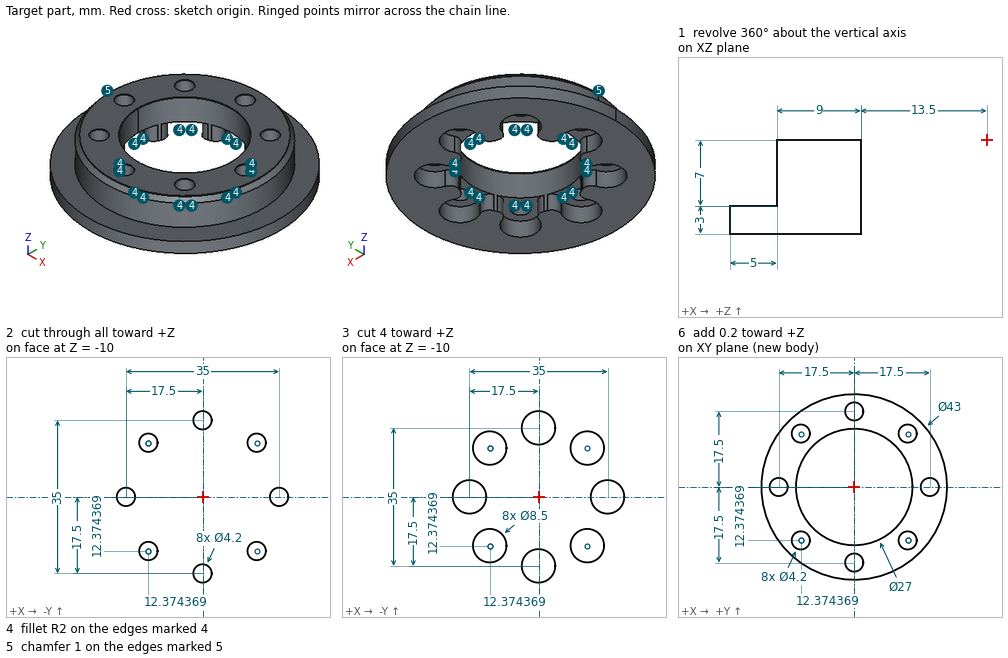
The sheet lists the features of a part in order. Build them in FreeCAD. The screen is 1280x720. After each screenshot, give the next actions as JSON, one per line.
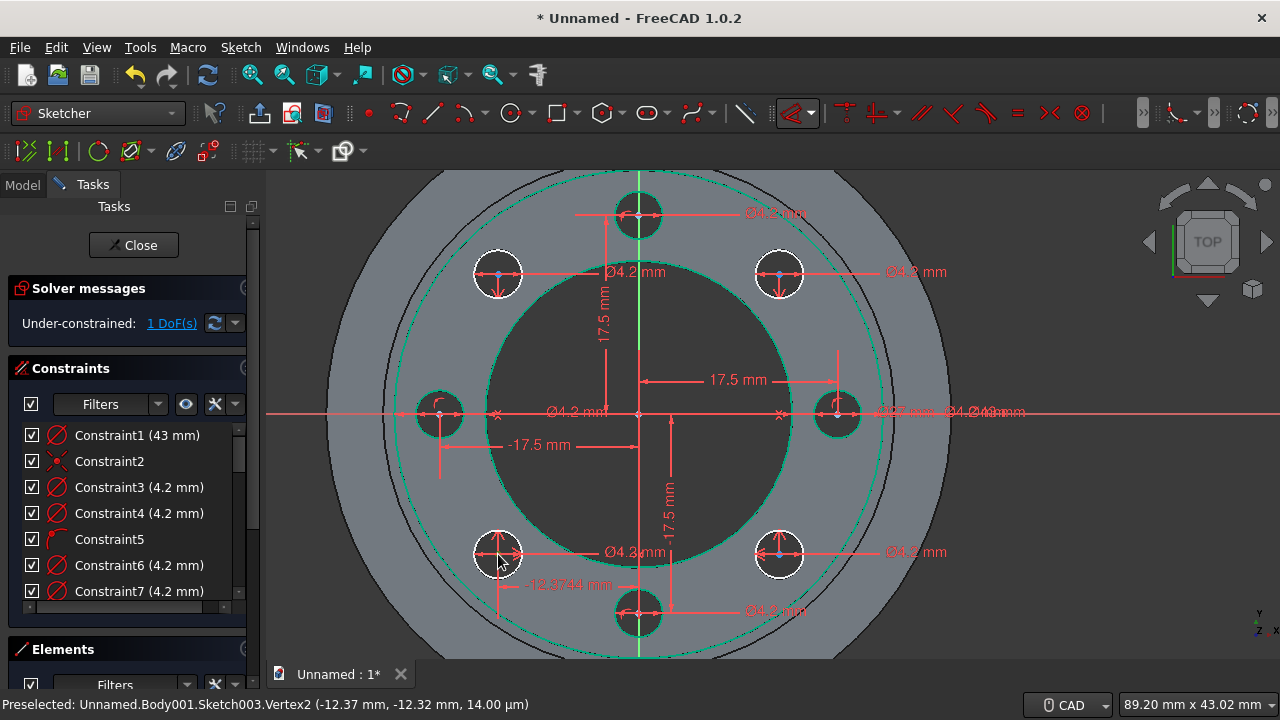
{"action": "key", "text": "i"}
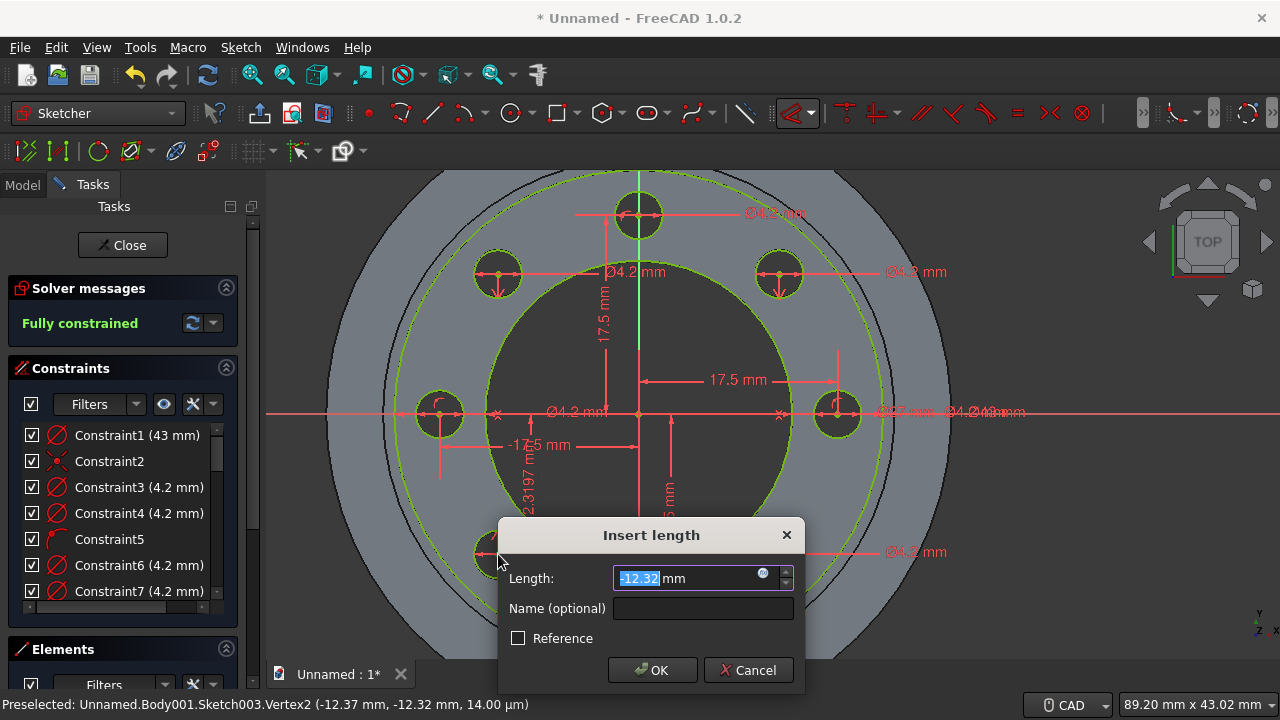
{"action": "type", "text": "-12.374369"}
{"action": "key", "text": "Return"}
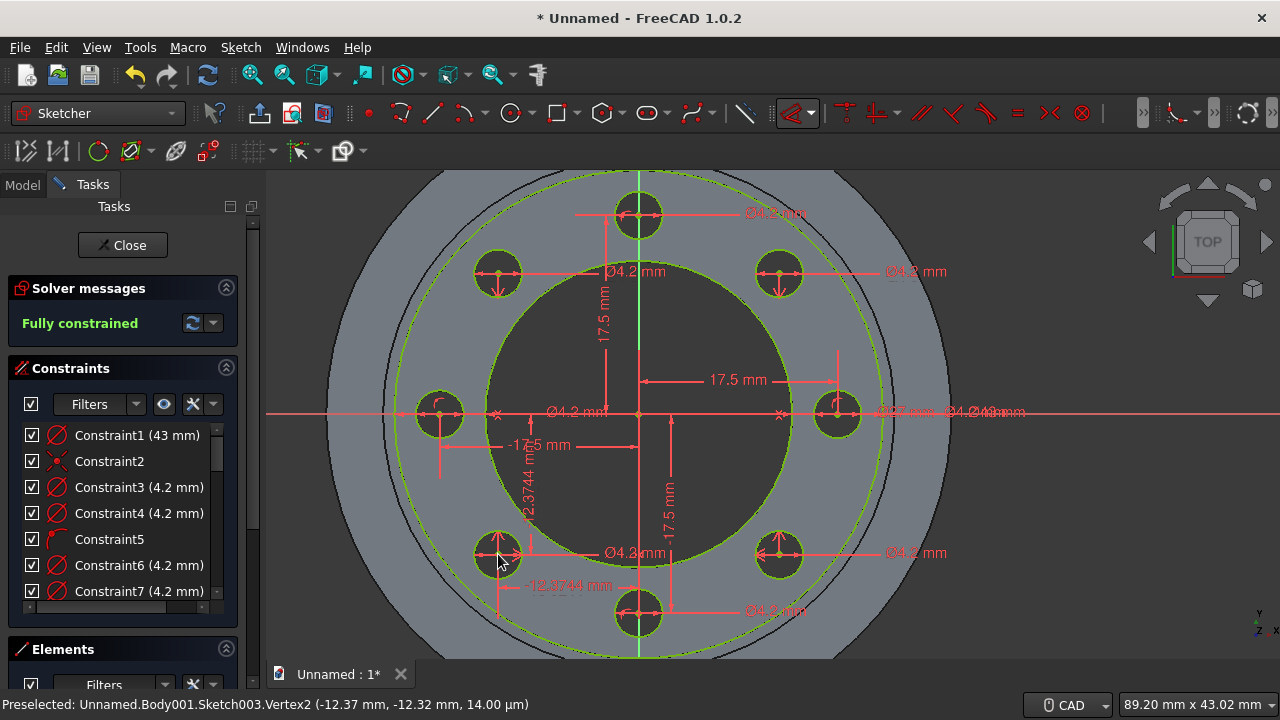
{"action": "left_click", "coordinate": [123, 245]}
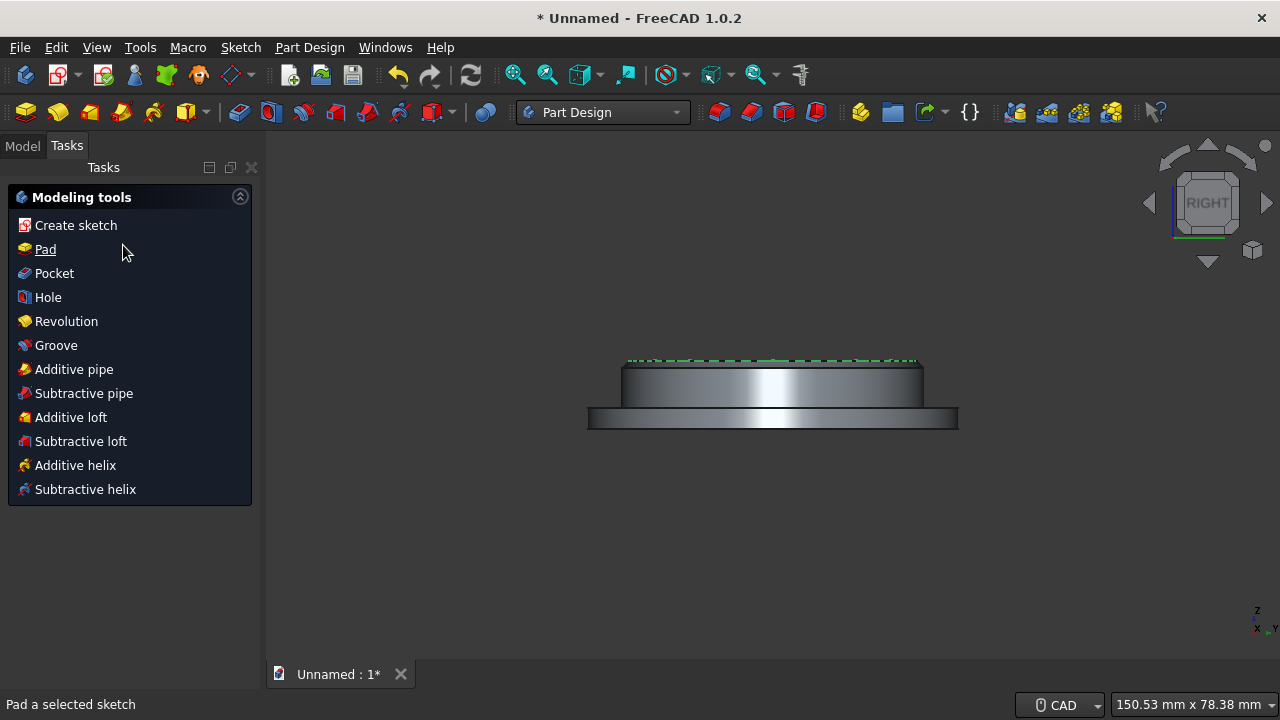
{"action": "left_click", "coordinate": [26, 112]}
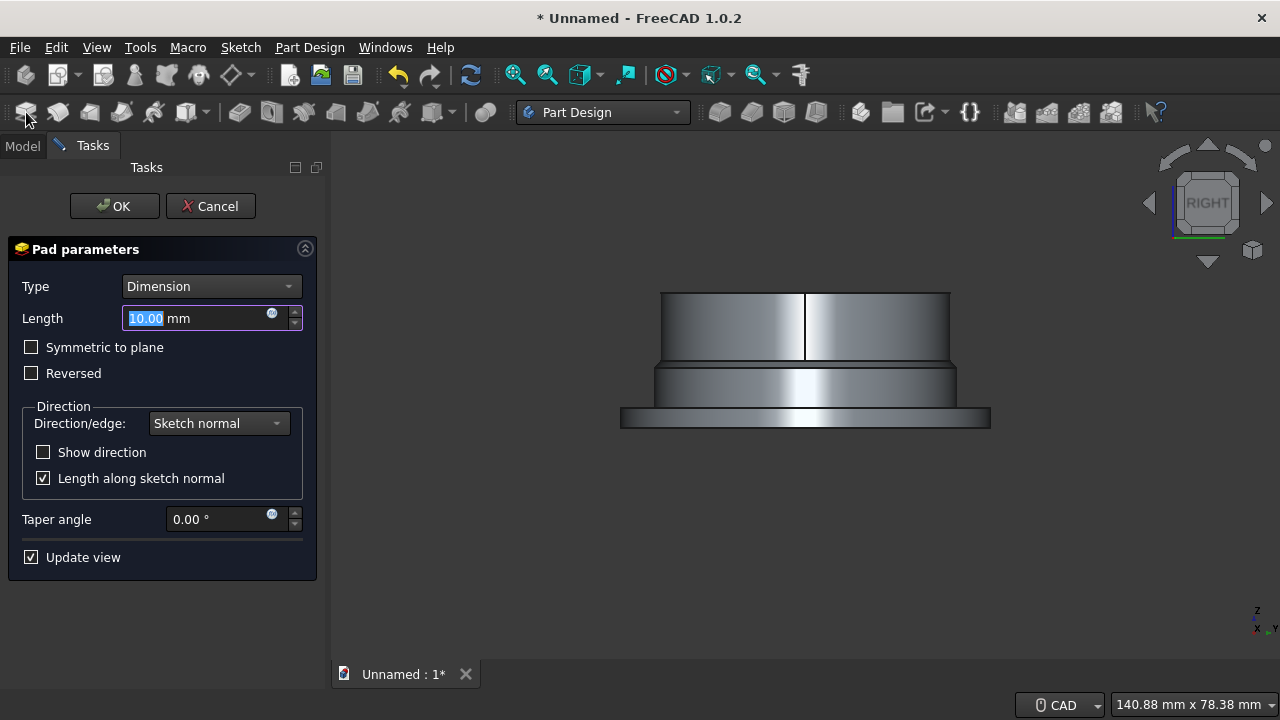
{"action": "type", "text": "0.2"}
{"action": "key", "text": "Tab"}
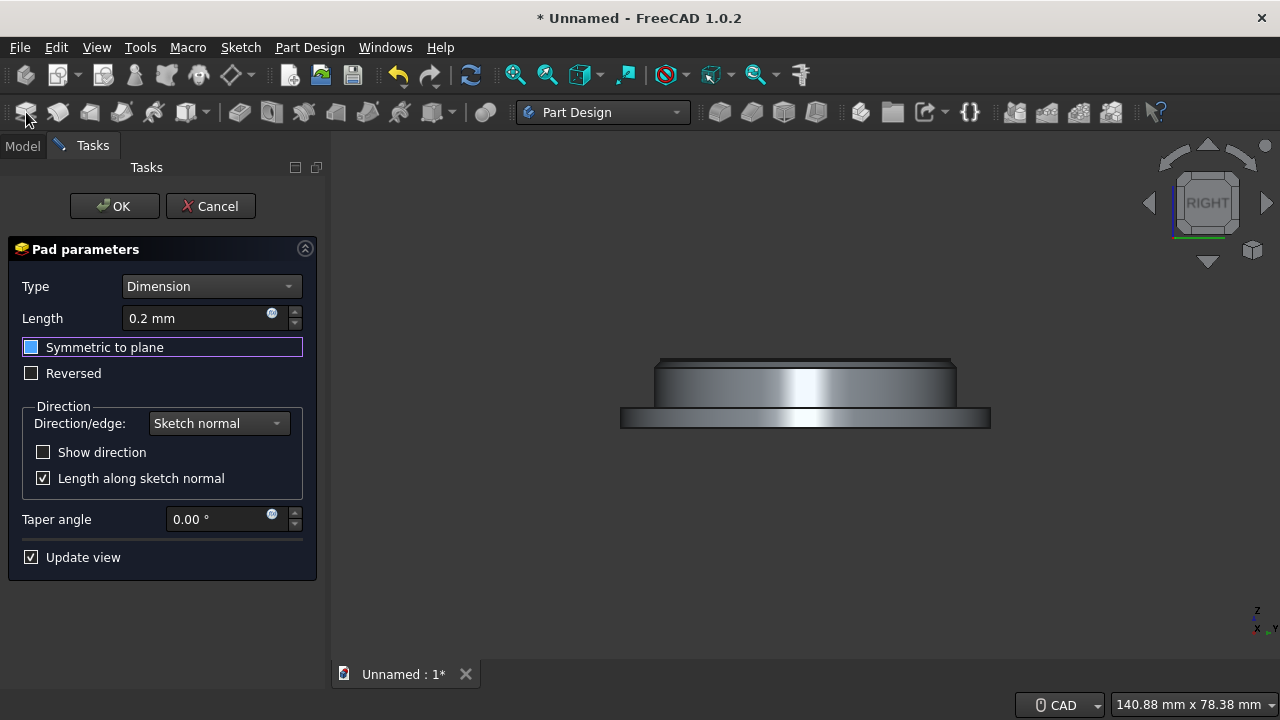
{"action": "left_click", "coordinate": [115, 206]}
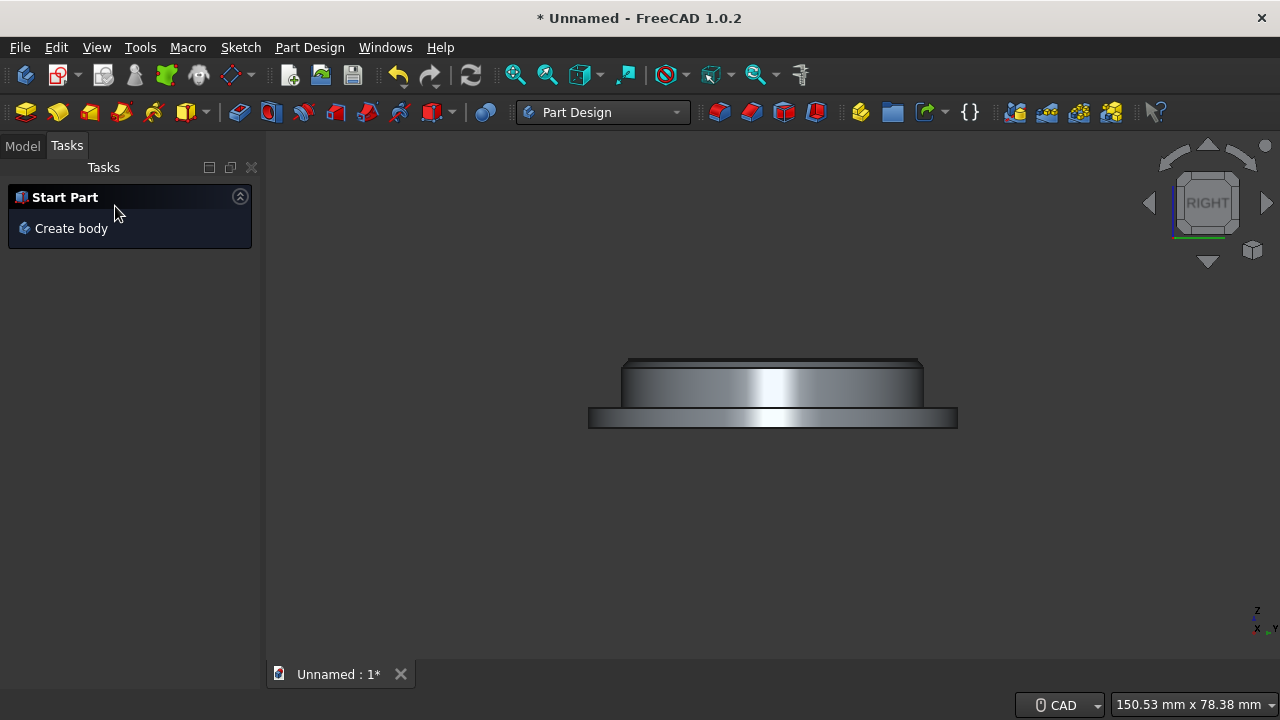
{"action": "key", "text": "0"}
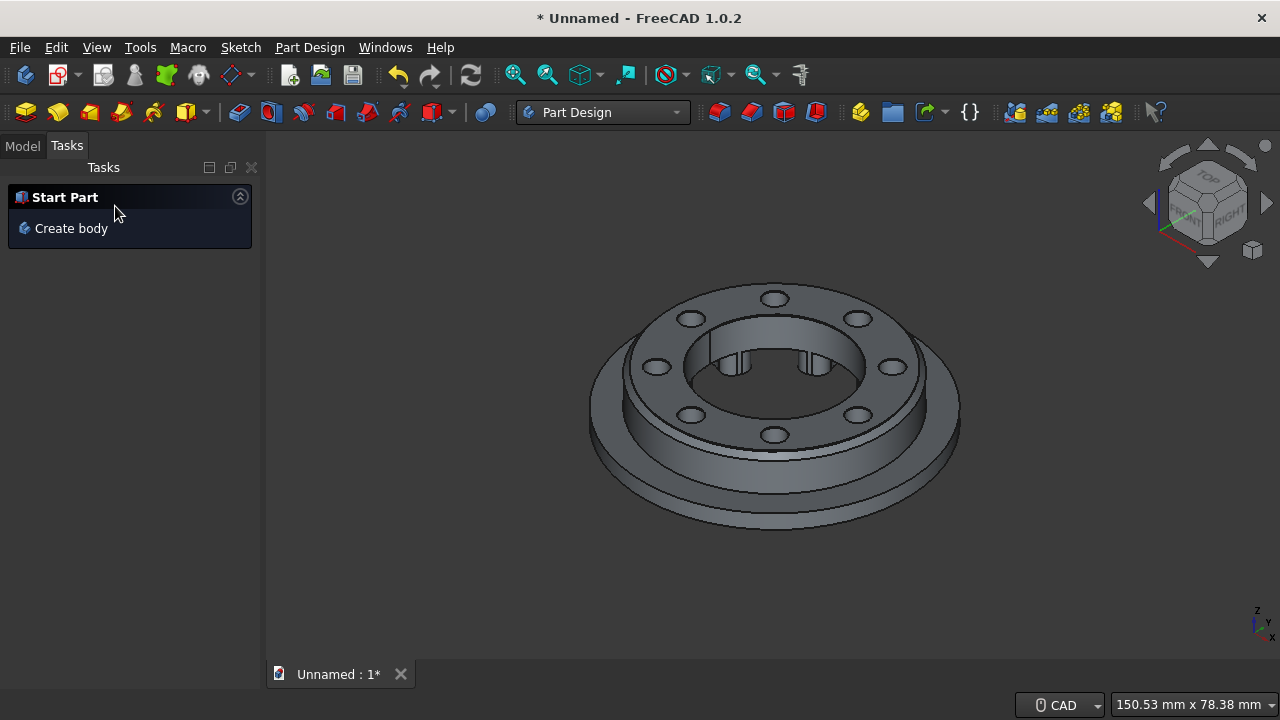
{"action": "key", "text": "v f"}